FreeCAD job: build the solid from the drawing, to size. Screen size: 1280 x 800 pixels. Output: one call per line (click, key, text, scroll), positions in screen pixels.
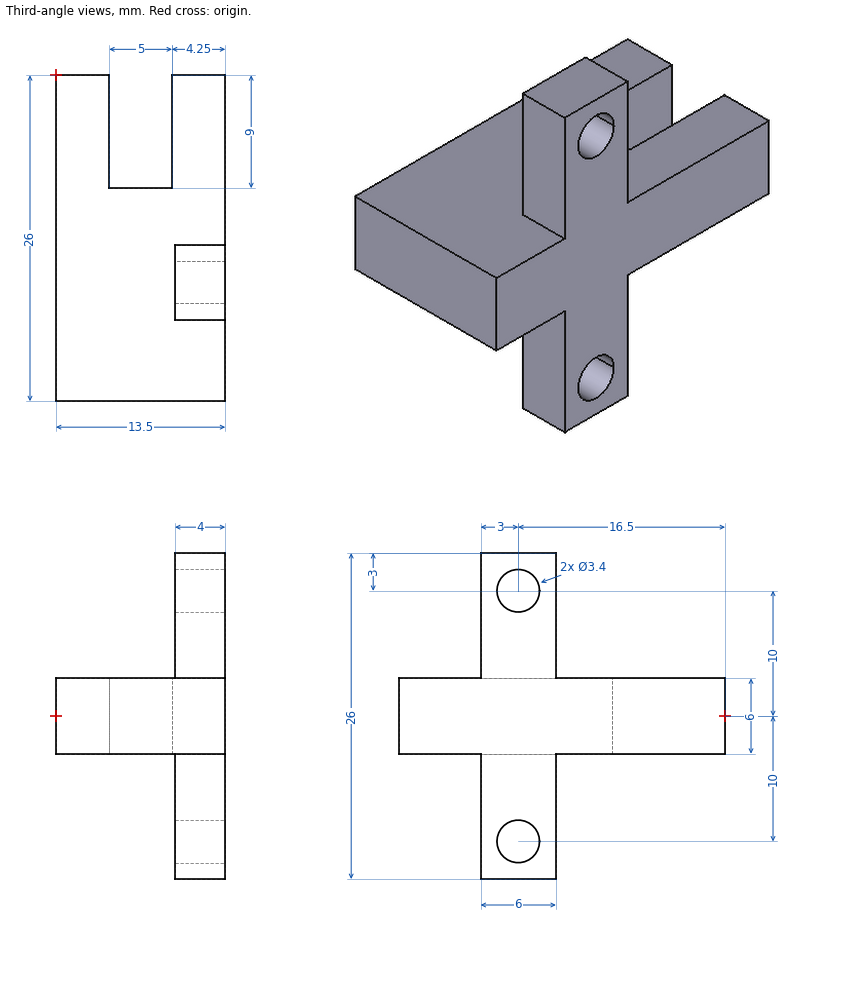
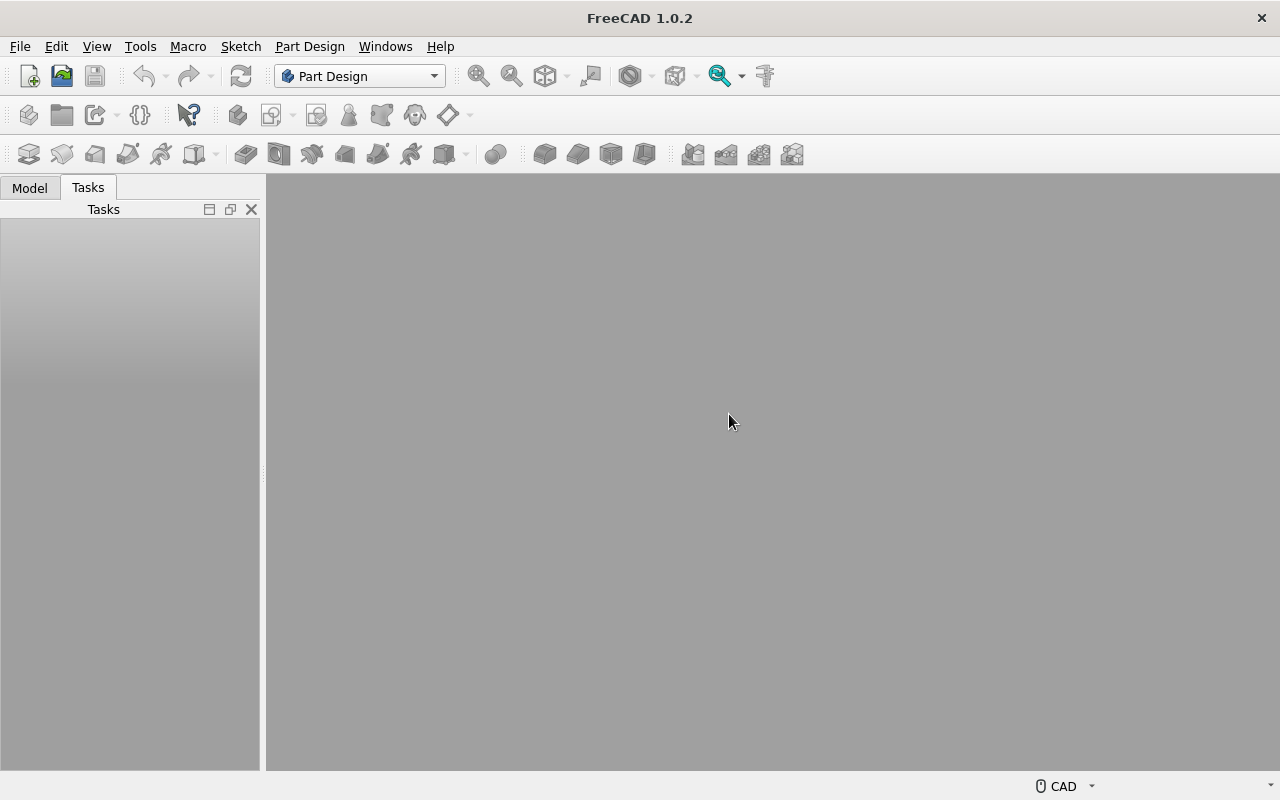
click(29, 76)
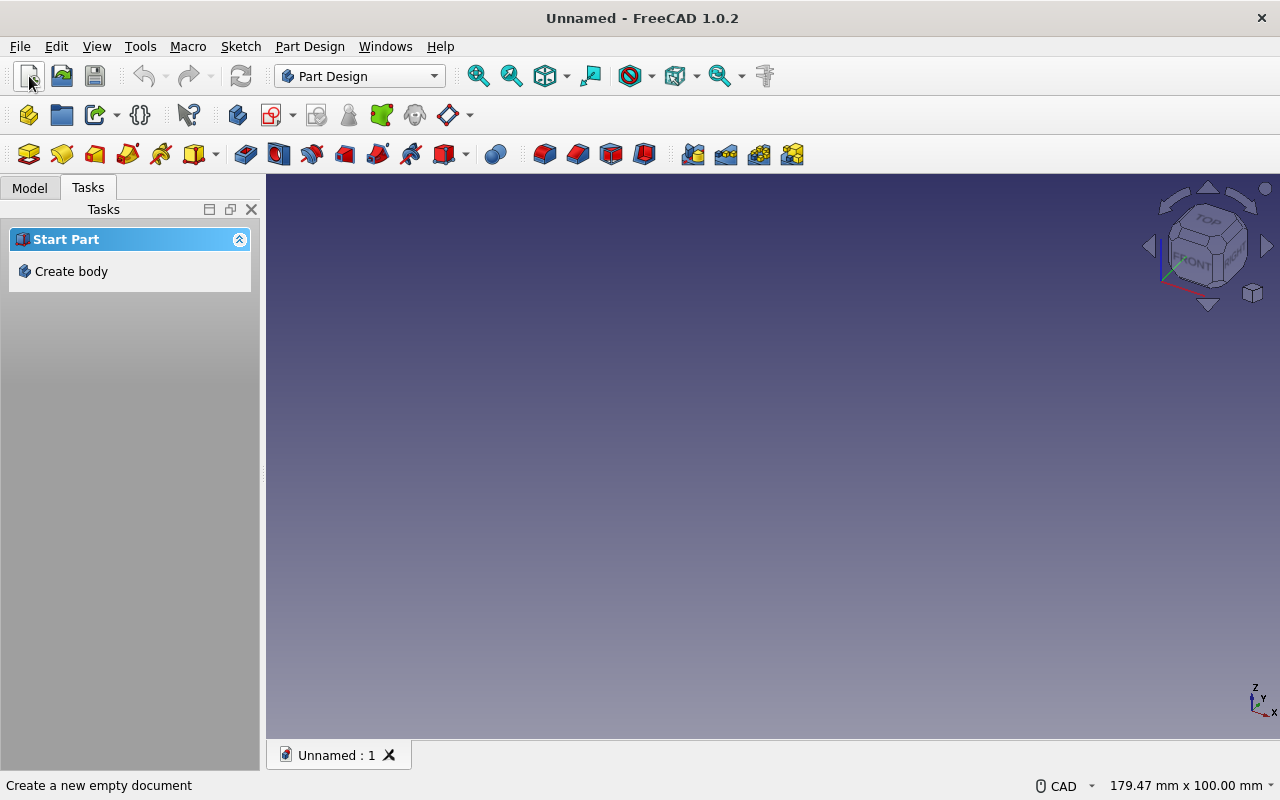
click(270, 116)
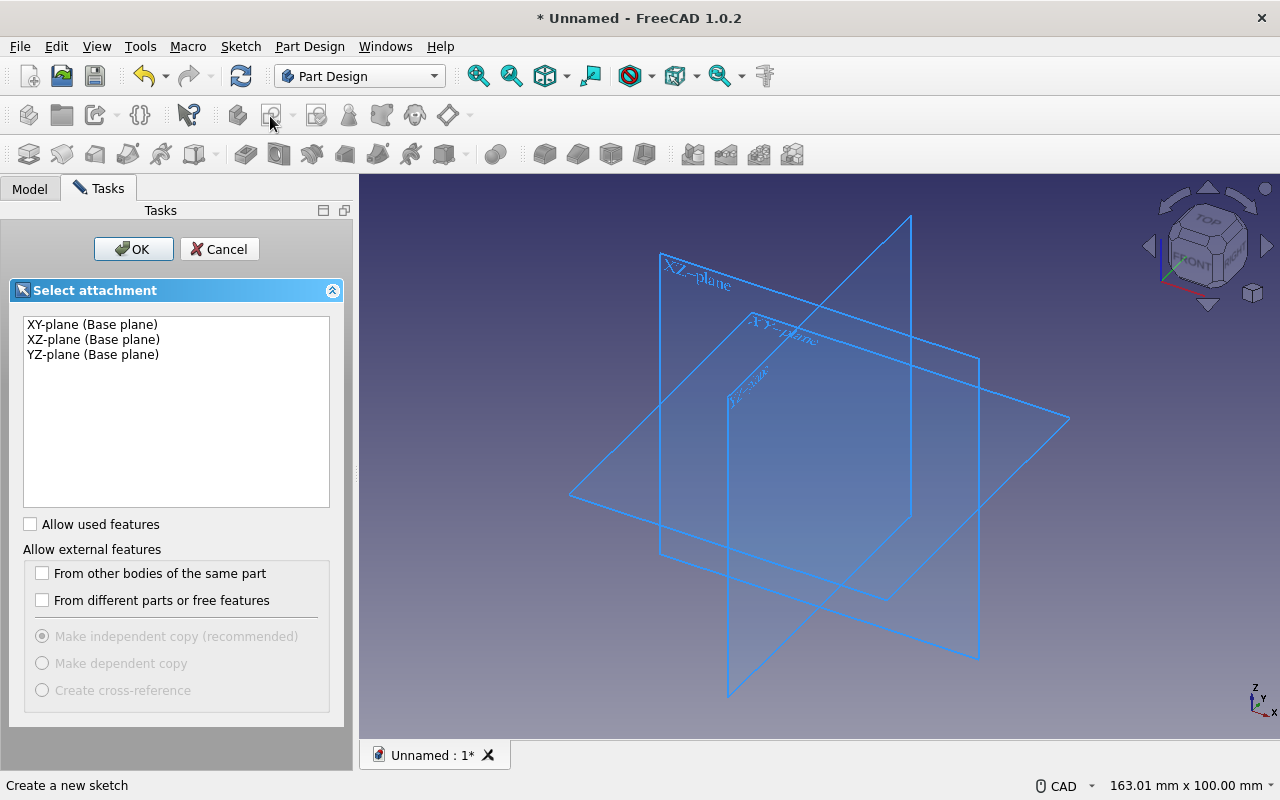
click(84, 324)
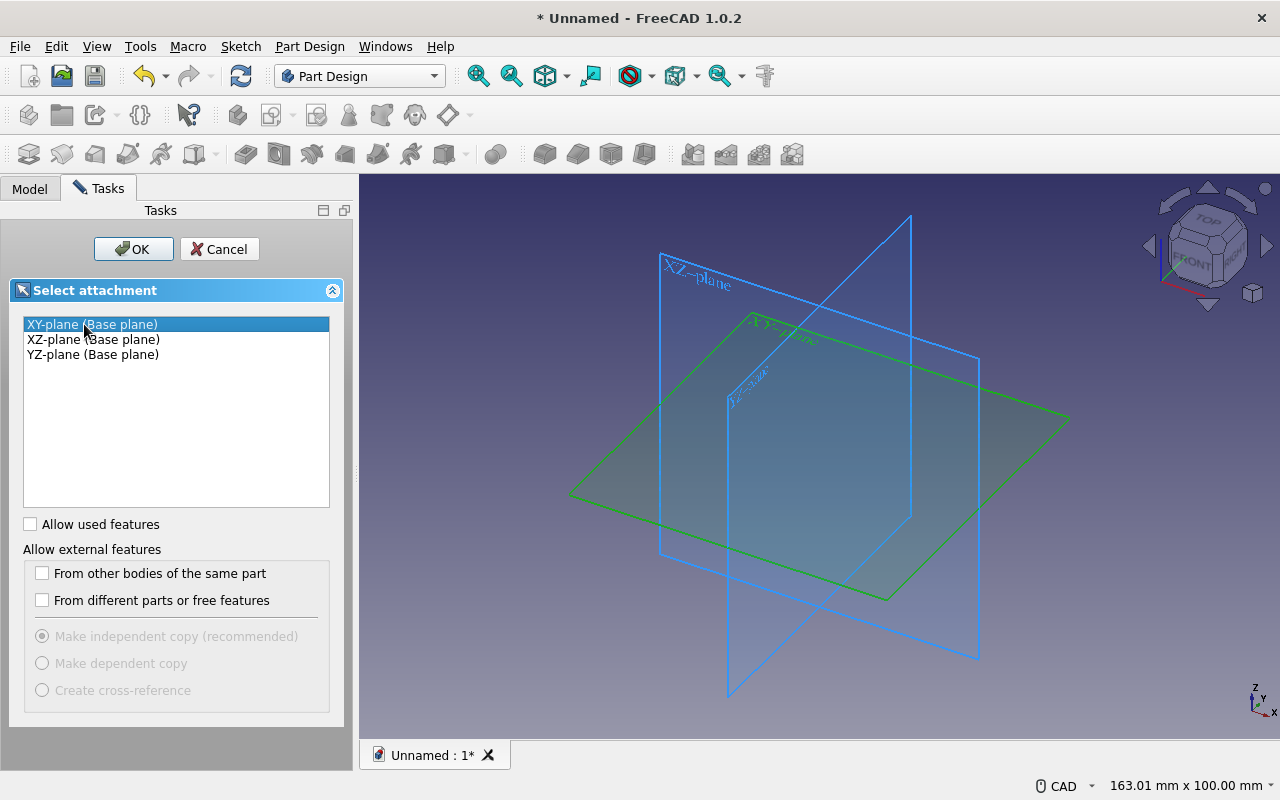
click(134, 249)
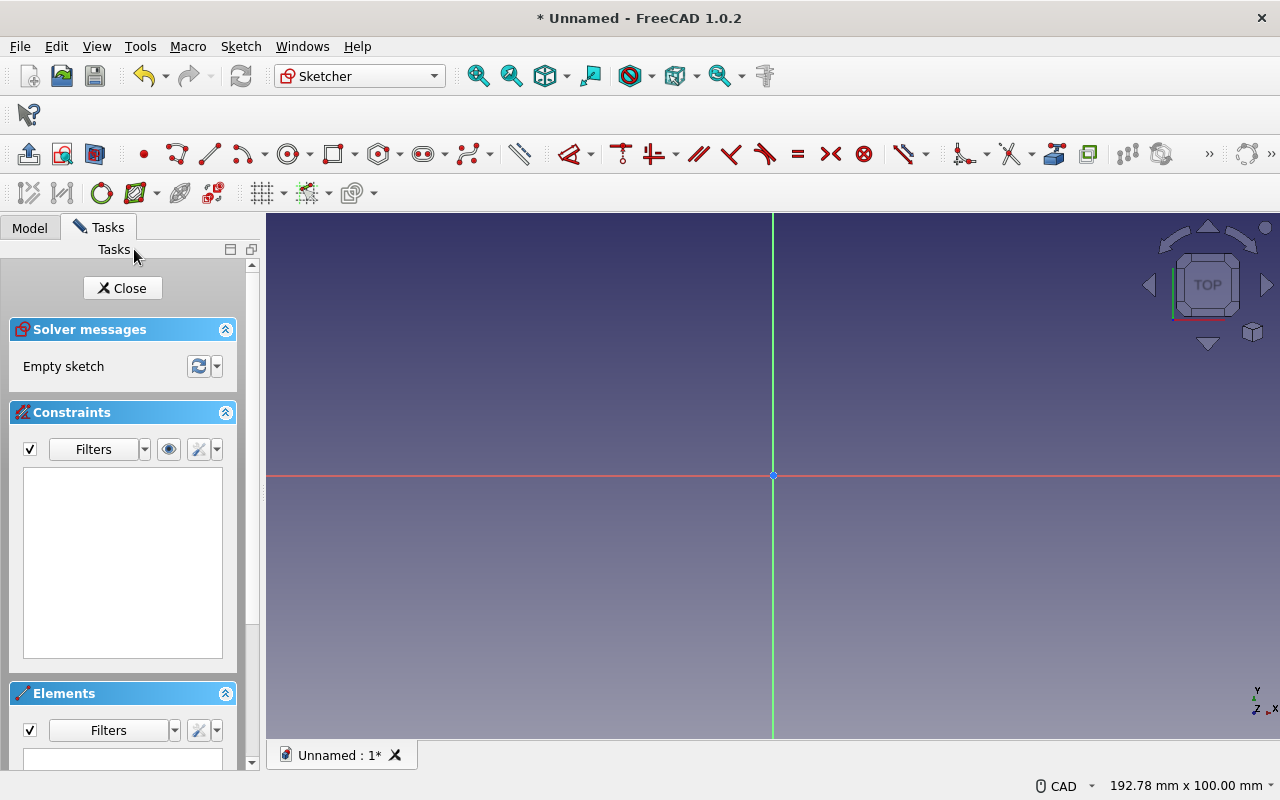
scroll(893, 600, up, 4)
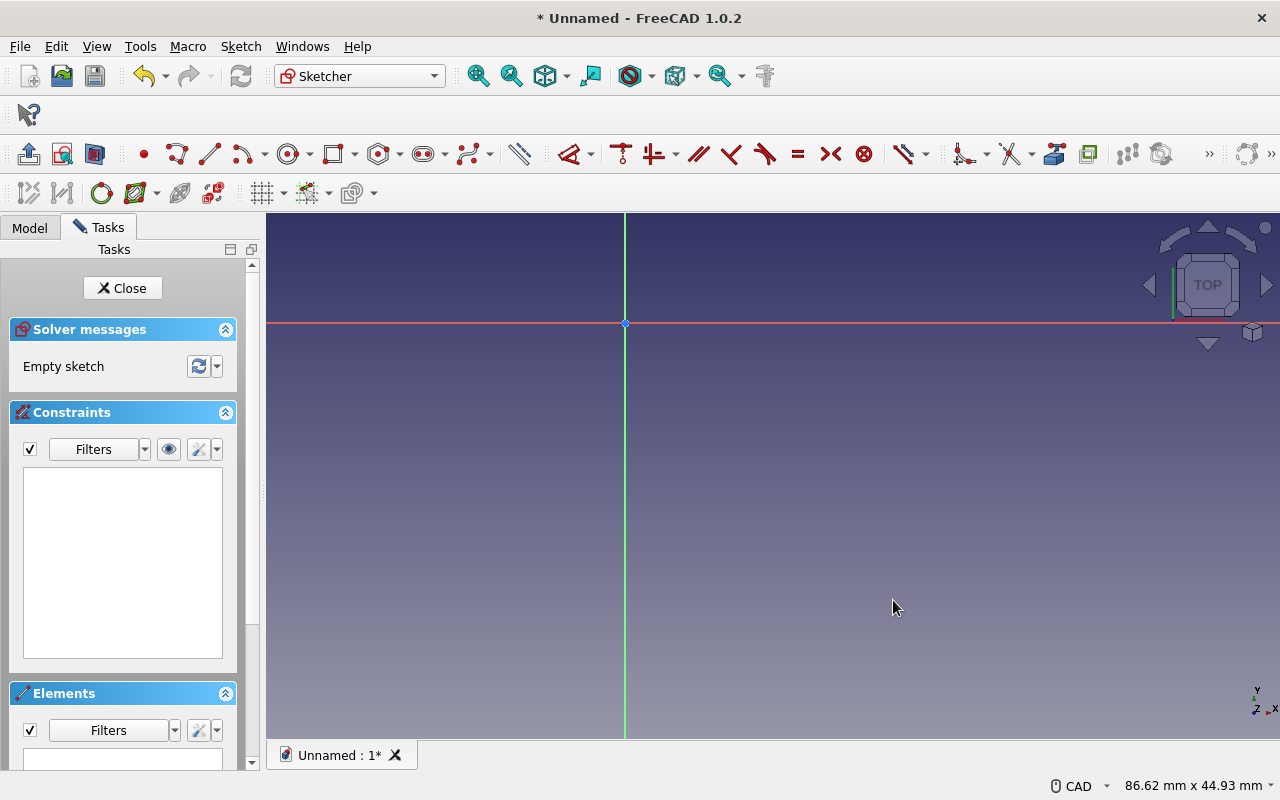
click(177, 154)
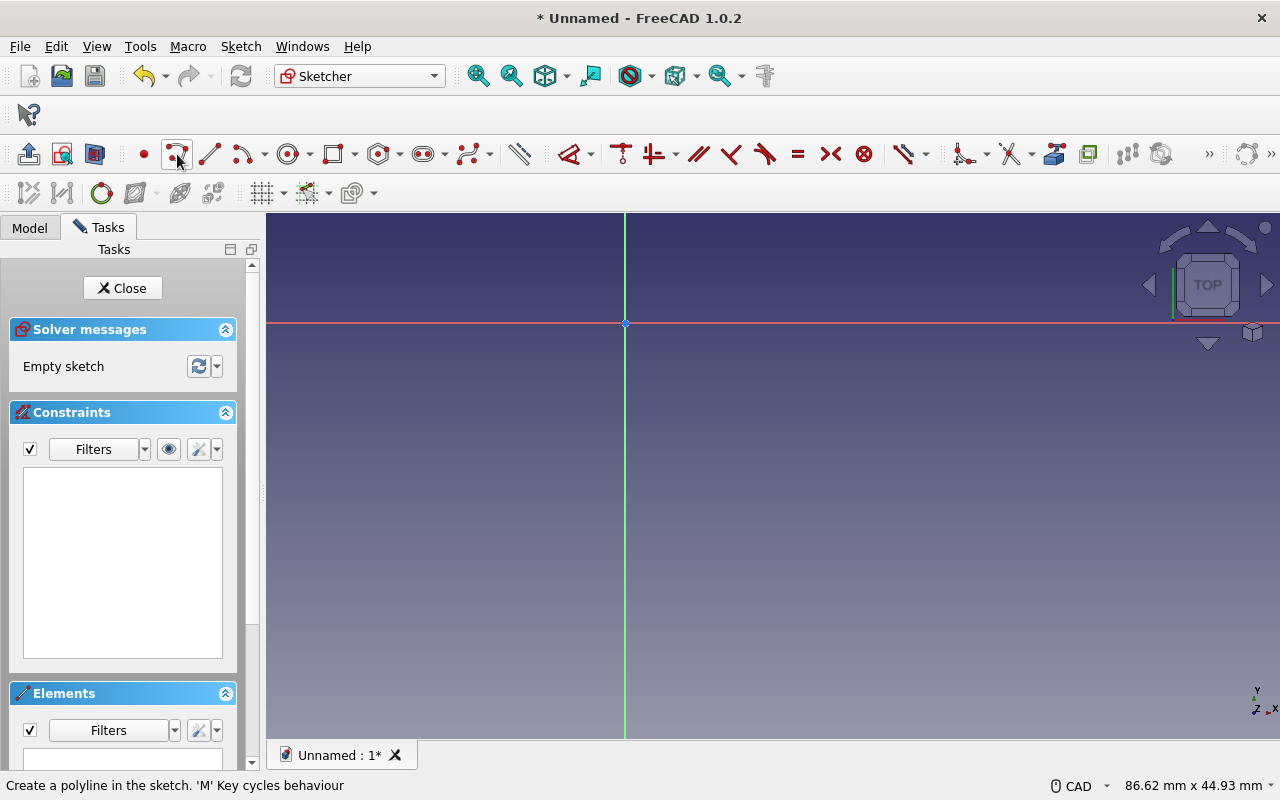
click(625, 323)
click(634, 627)
click(783, 627)
click(783, 323)
click(733, 332)
click(733, 428)
click(675, 428)
click(675, 332)
click(625, 323)
key(Escape)
key(Escape)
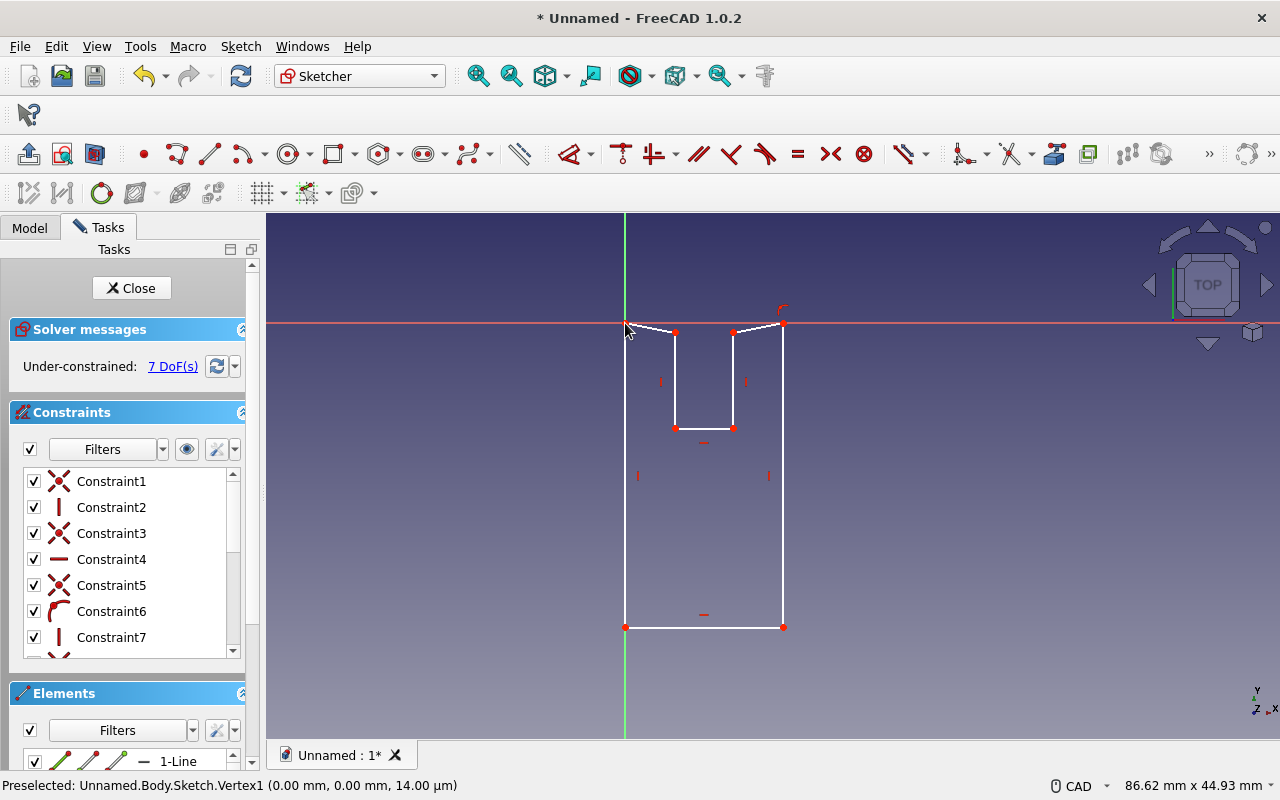
click(768, 326)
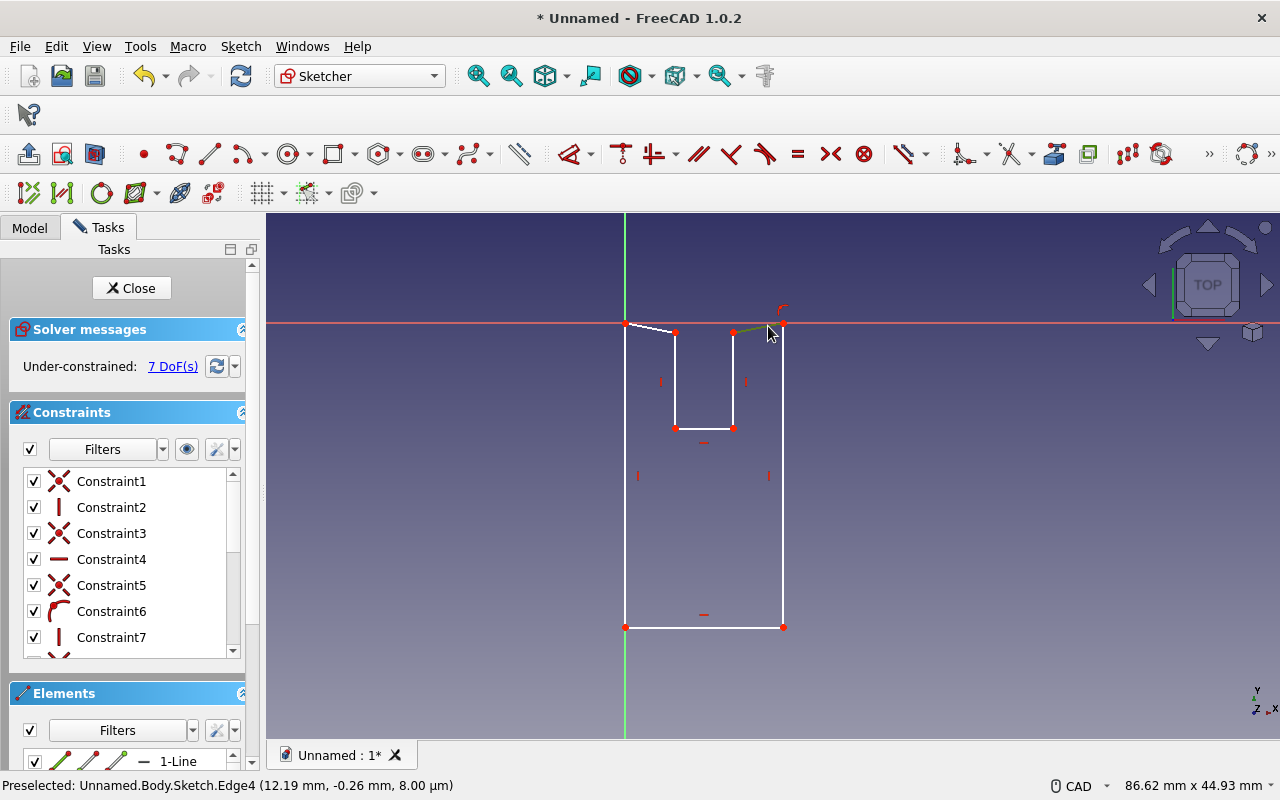
click(676, 154)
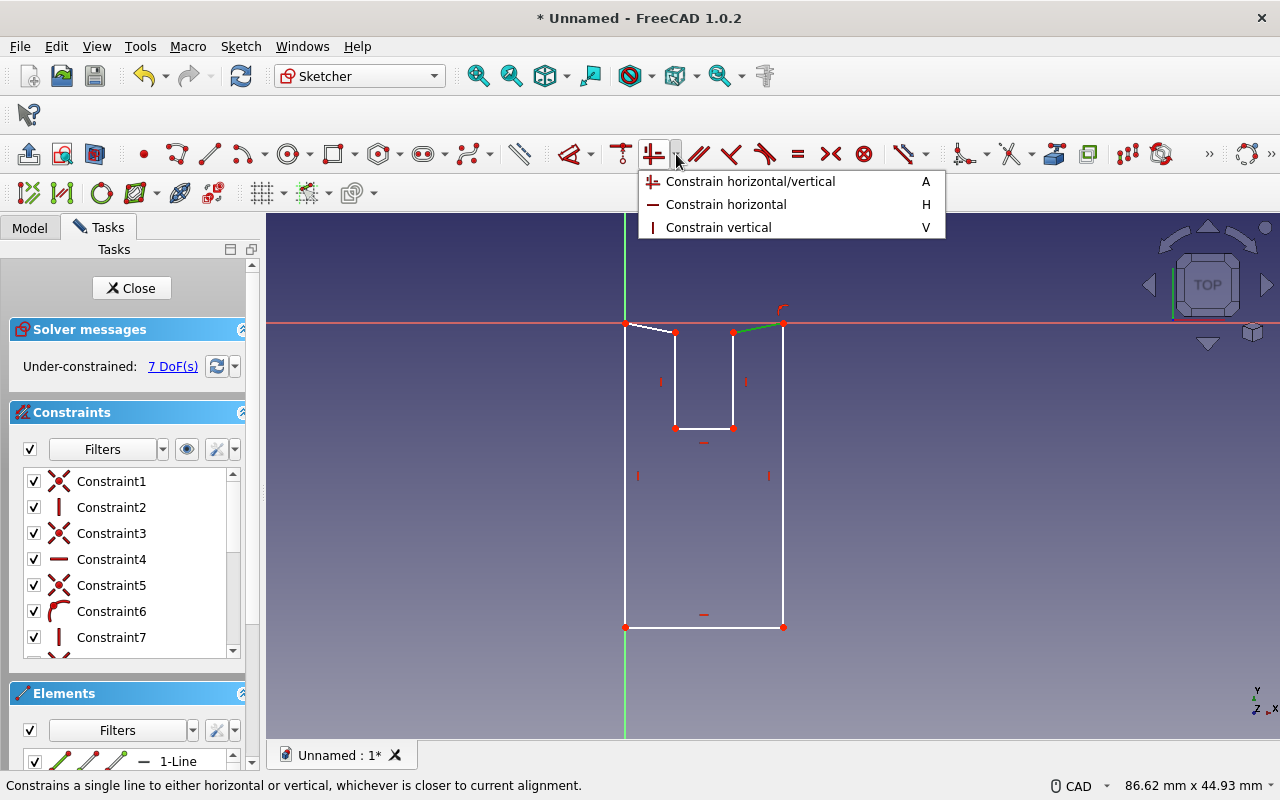
click(792, 204)